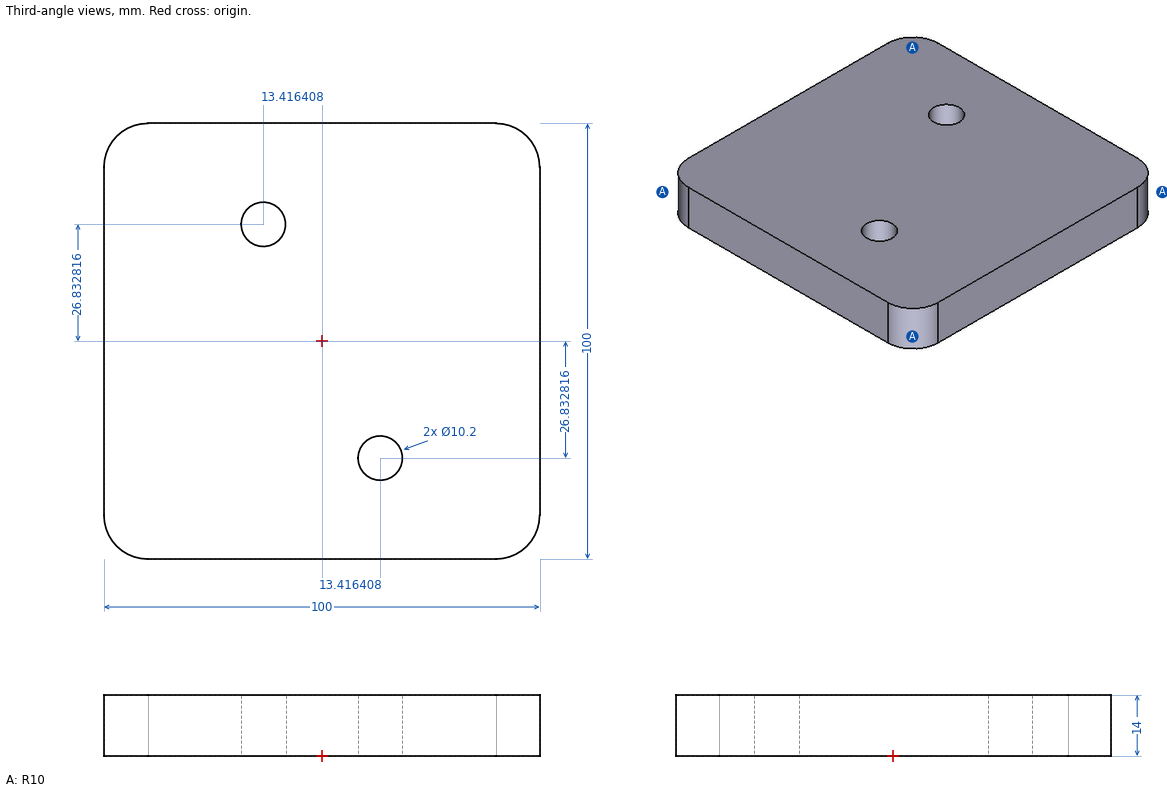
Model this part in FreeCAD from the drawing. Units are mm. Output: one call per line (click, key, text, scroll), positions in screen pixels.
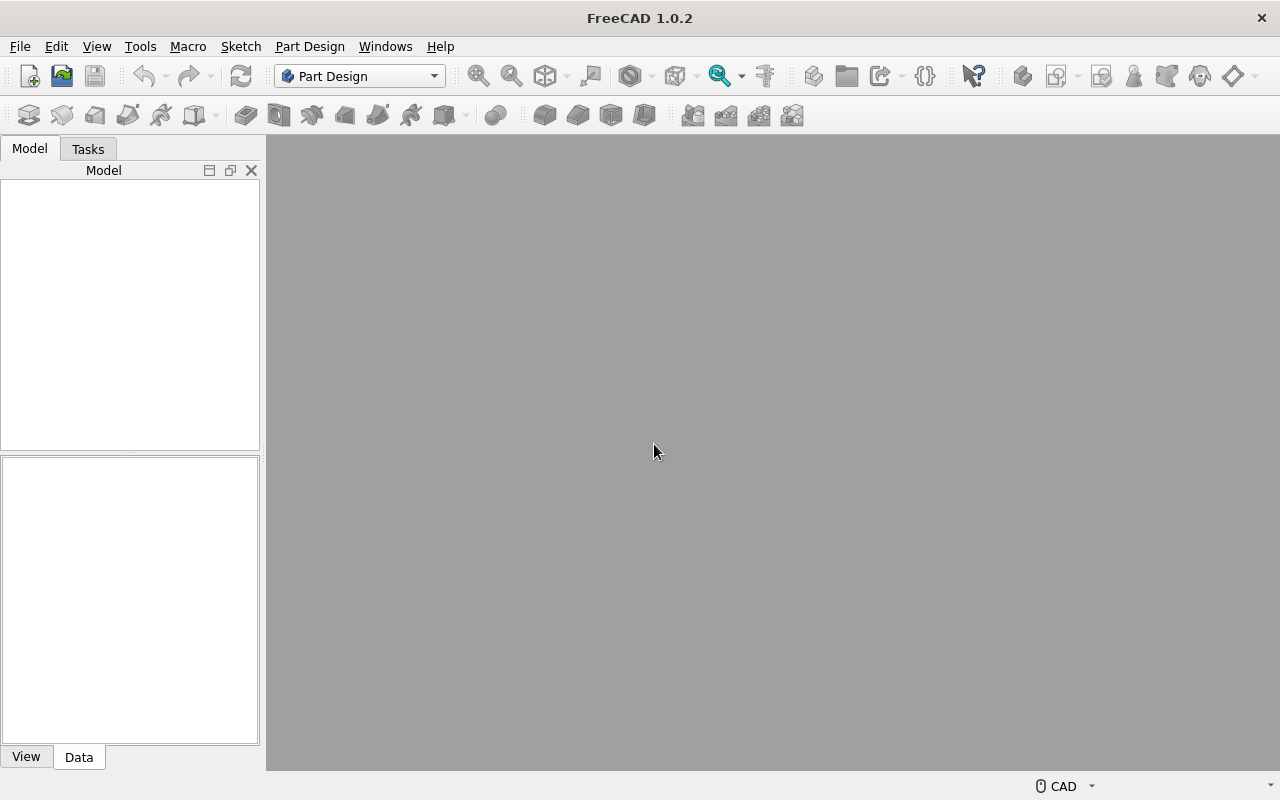
click(29, 76)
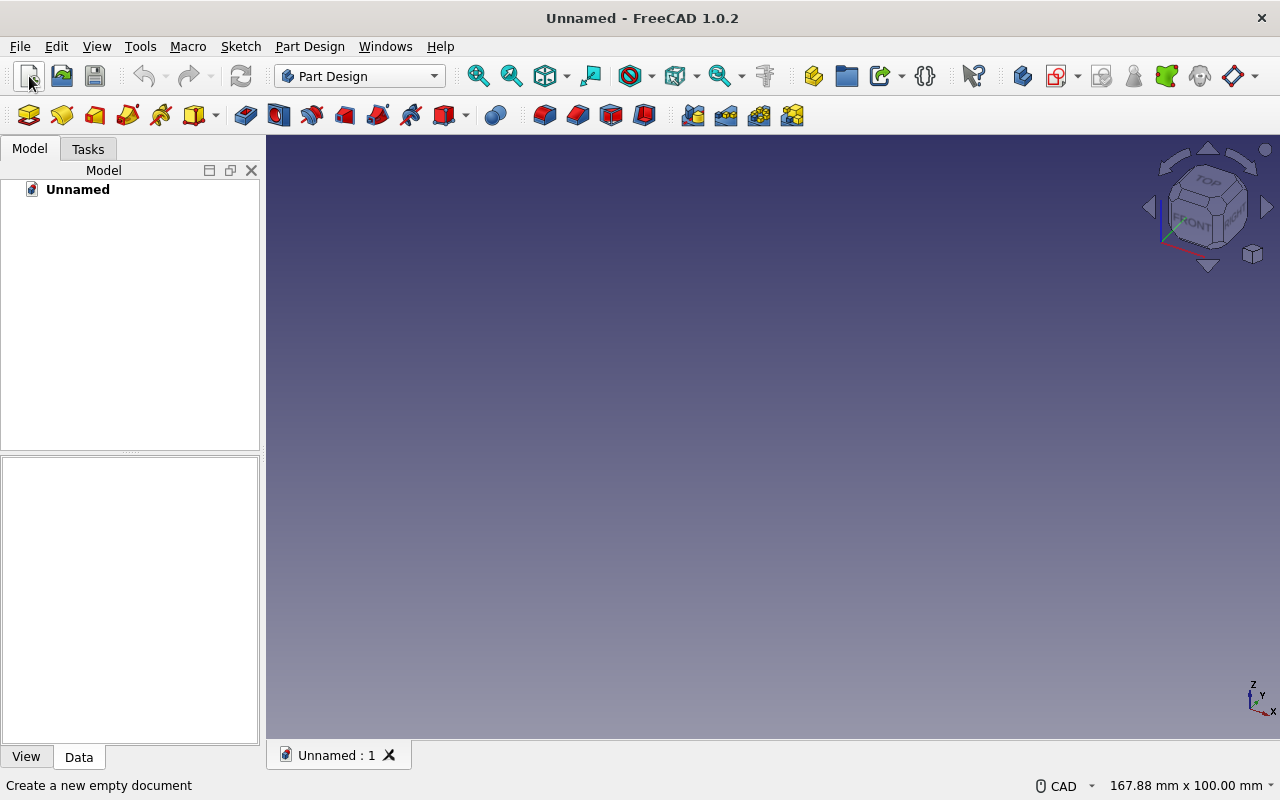
click(1056, 76)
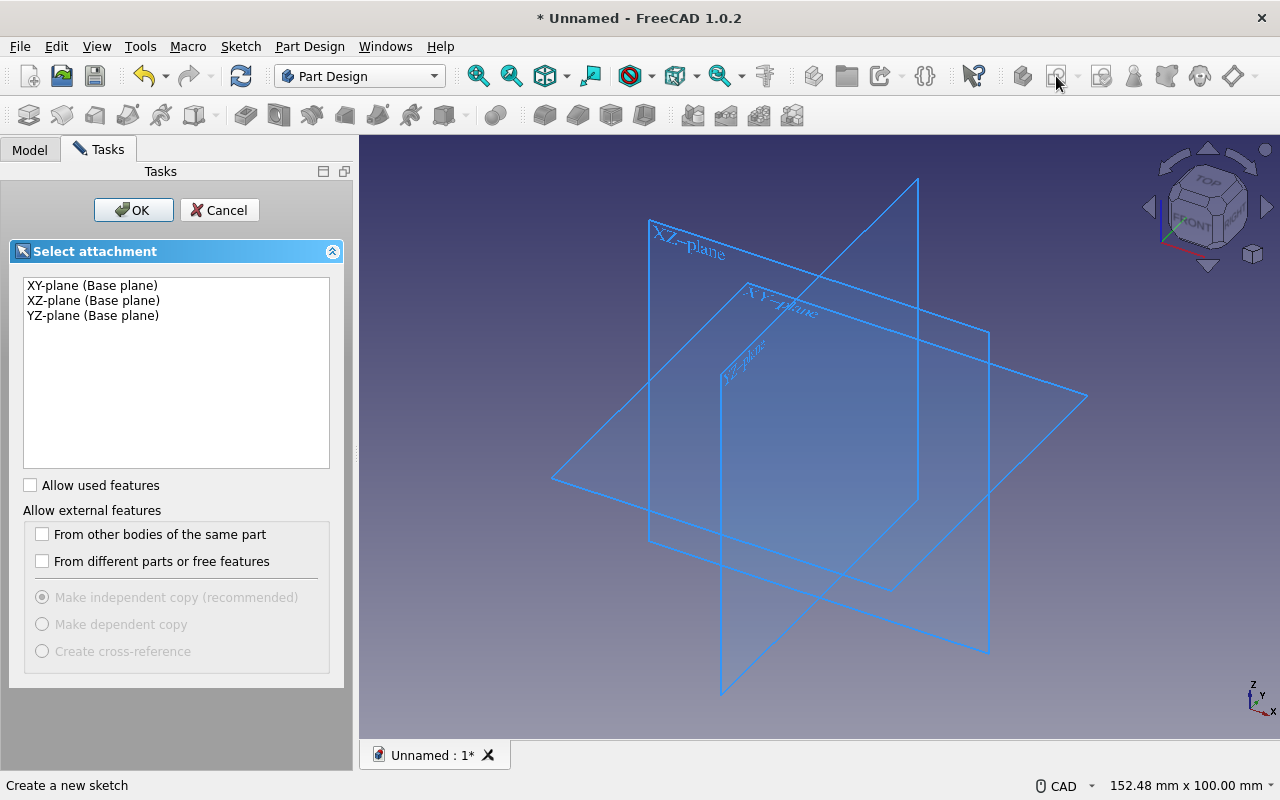
click(84, 286)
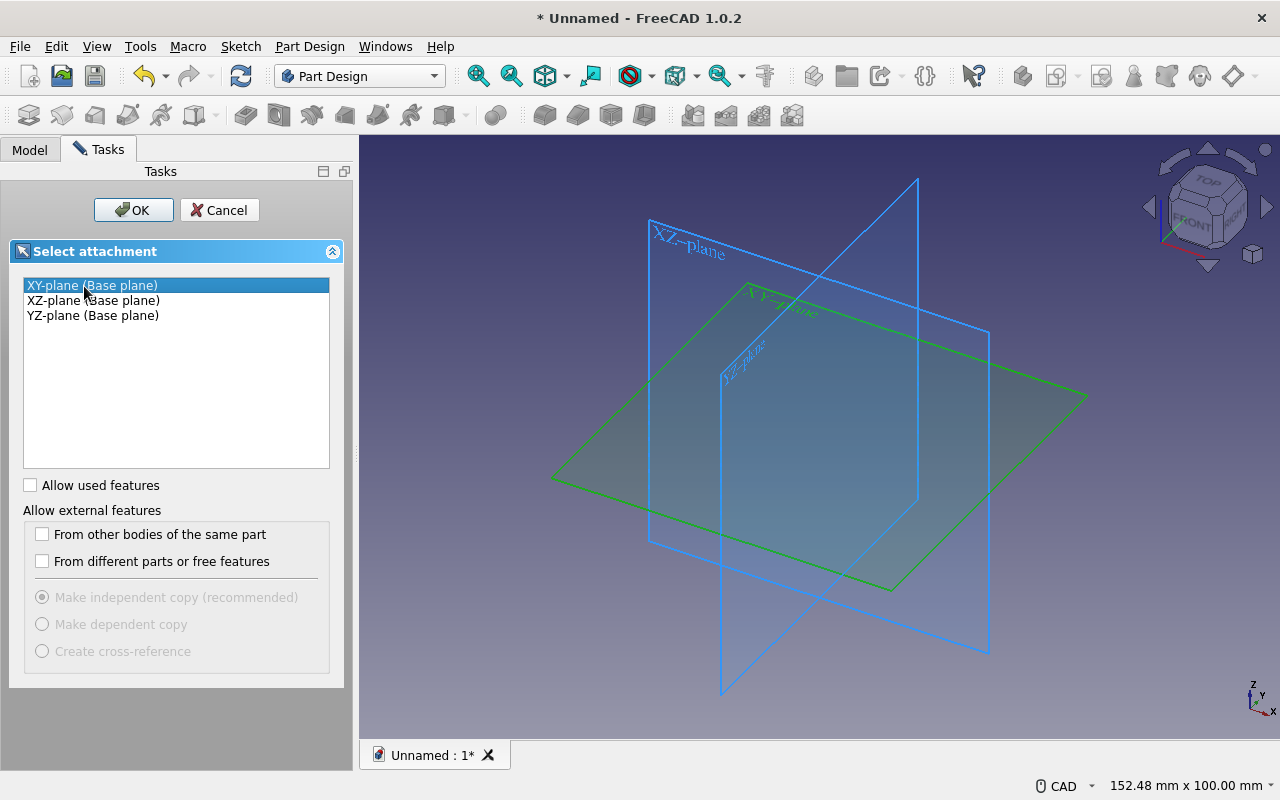
click(134, 210)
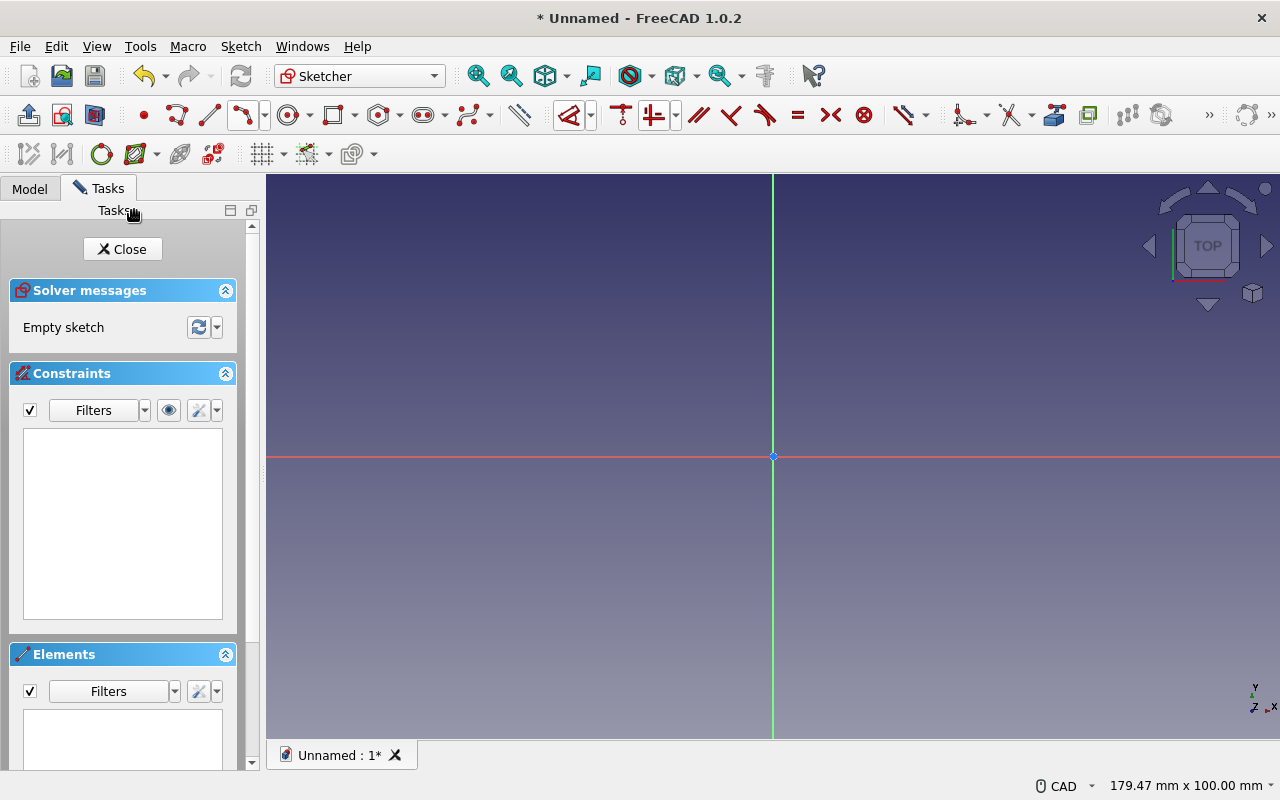
scroll(565, 457, down, 2)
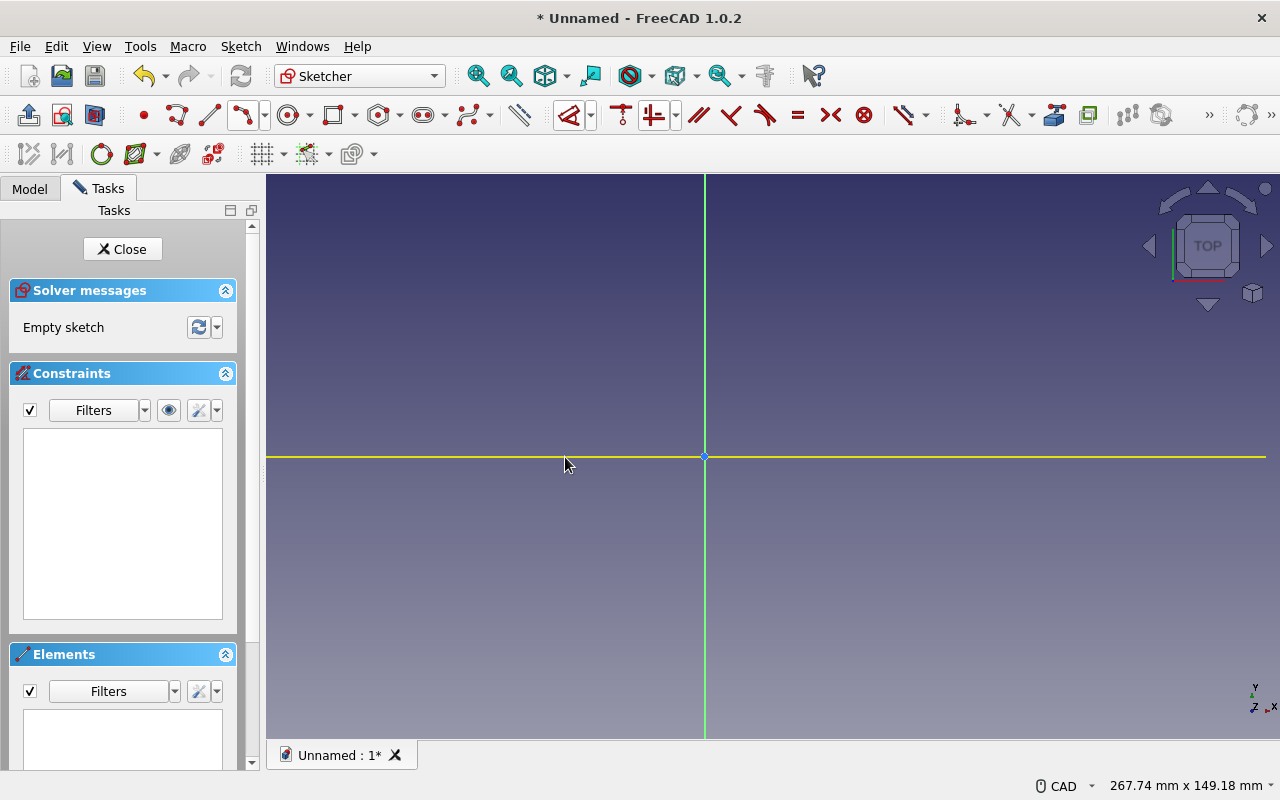
key(g)
key(v)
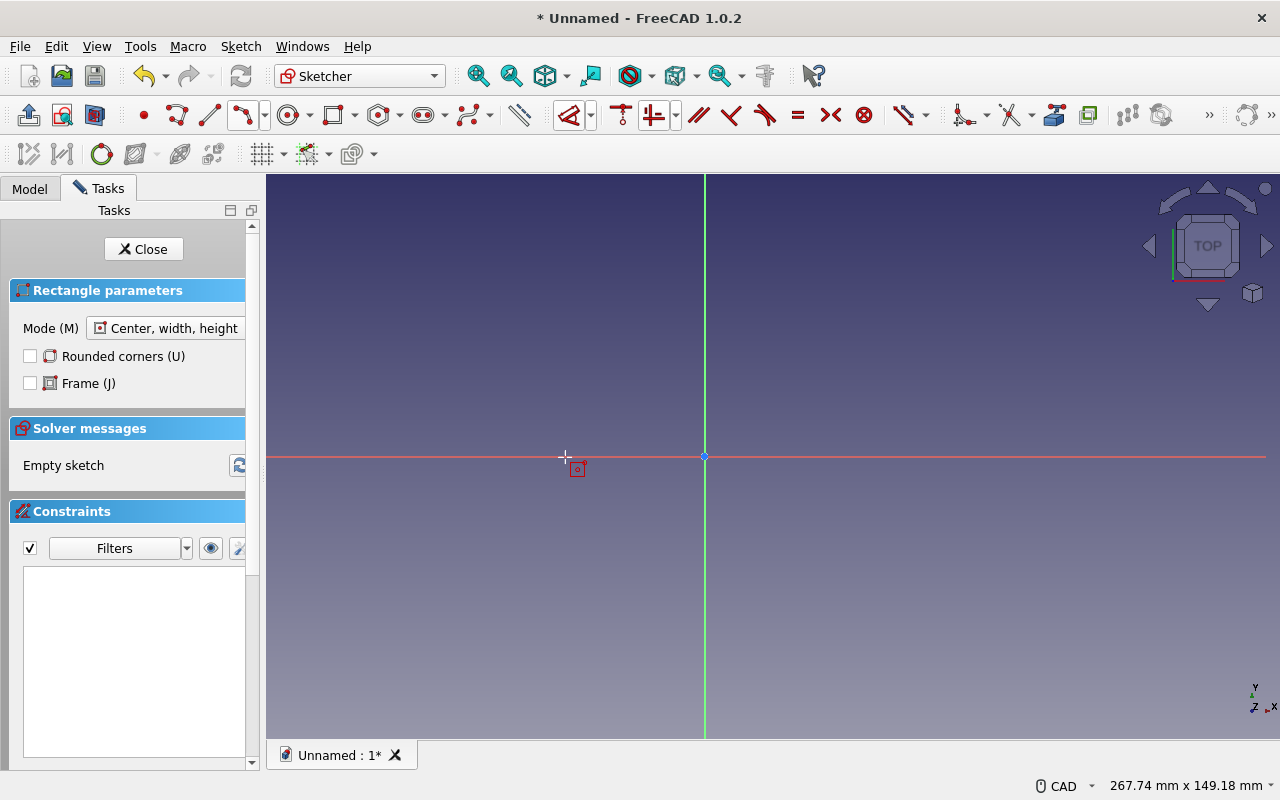
click(705, 457)
click(894, 267)
key(Escape)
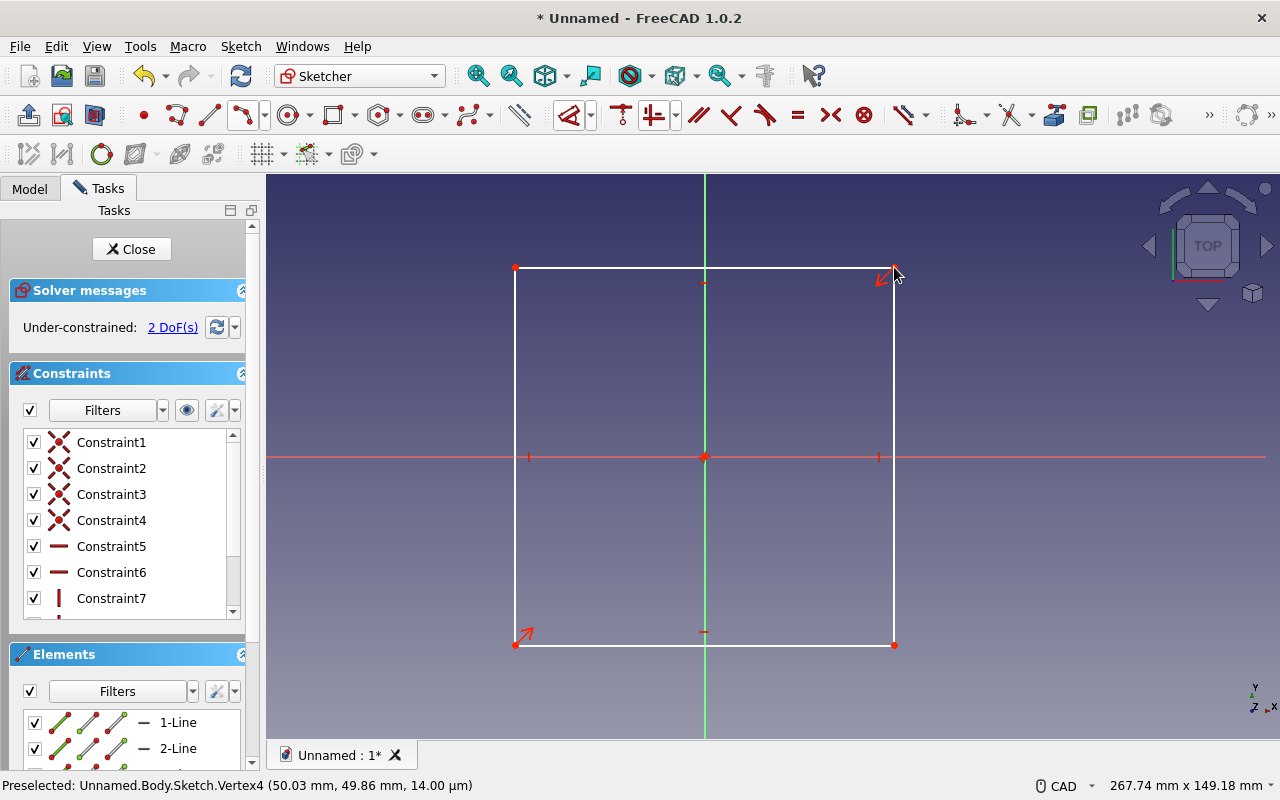
click(629, 646)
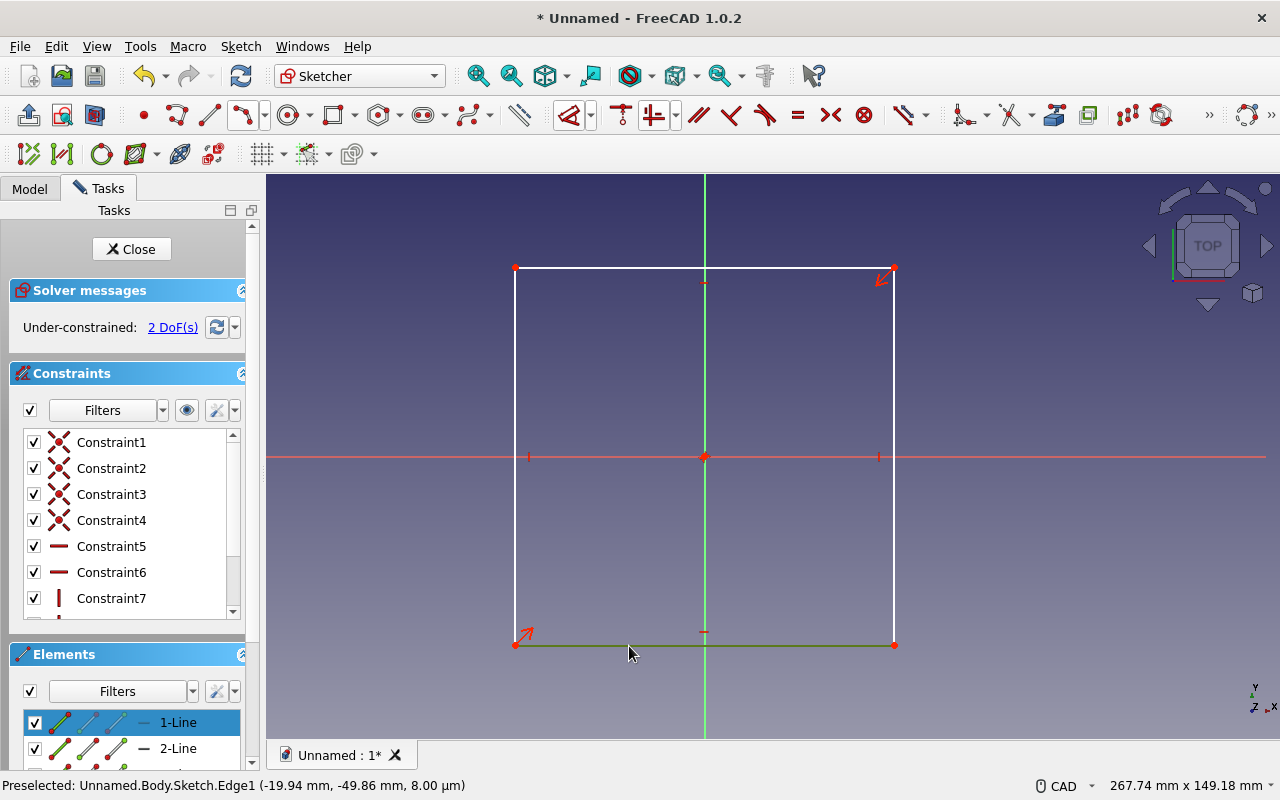
key(l)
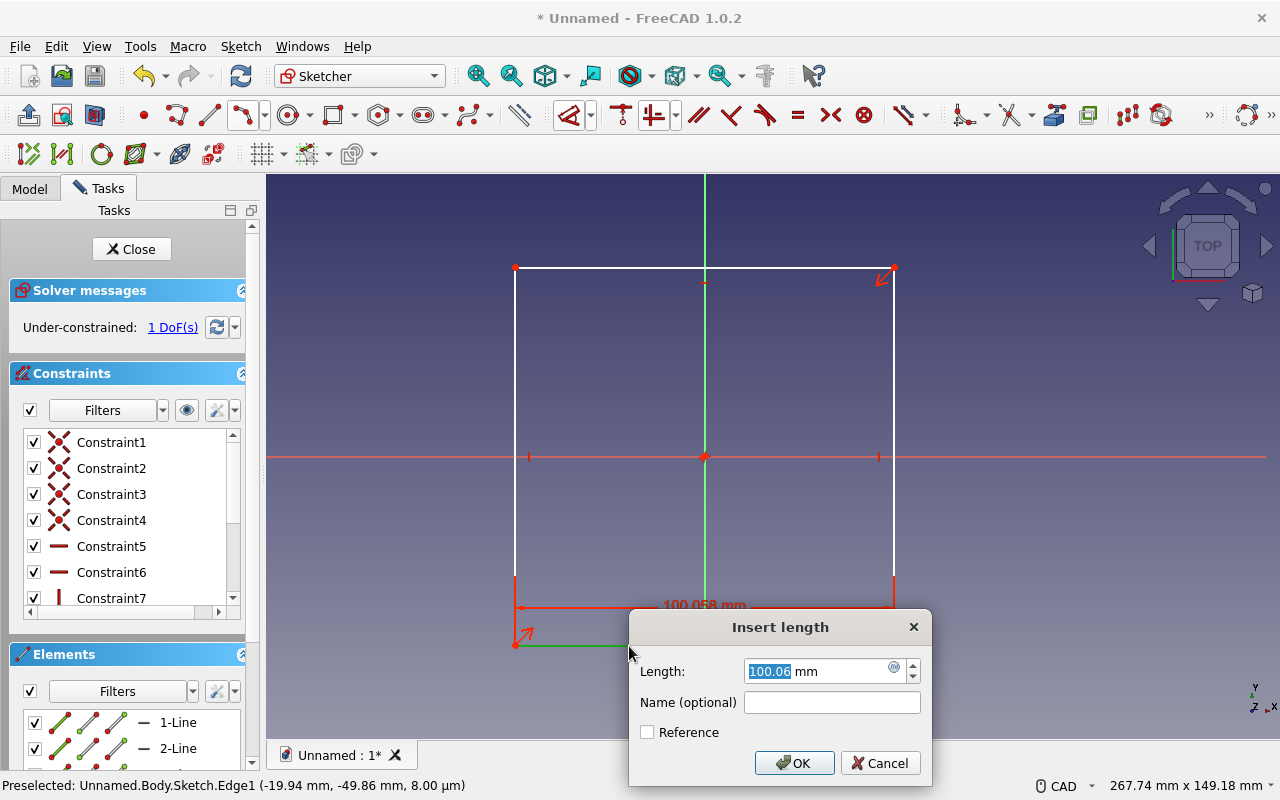
text(100)
key(Return)